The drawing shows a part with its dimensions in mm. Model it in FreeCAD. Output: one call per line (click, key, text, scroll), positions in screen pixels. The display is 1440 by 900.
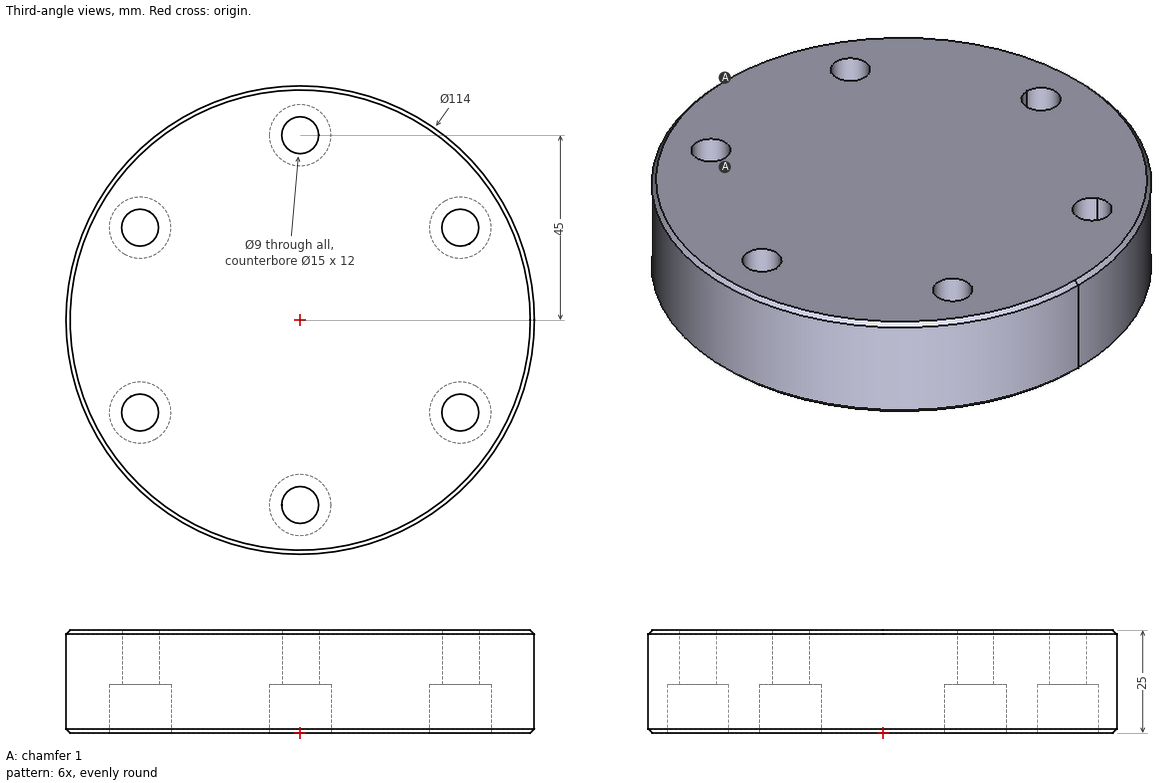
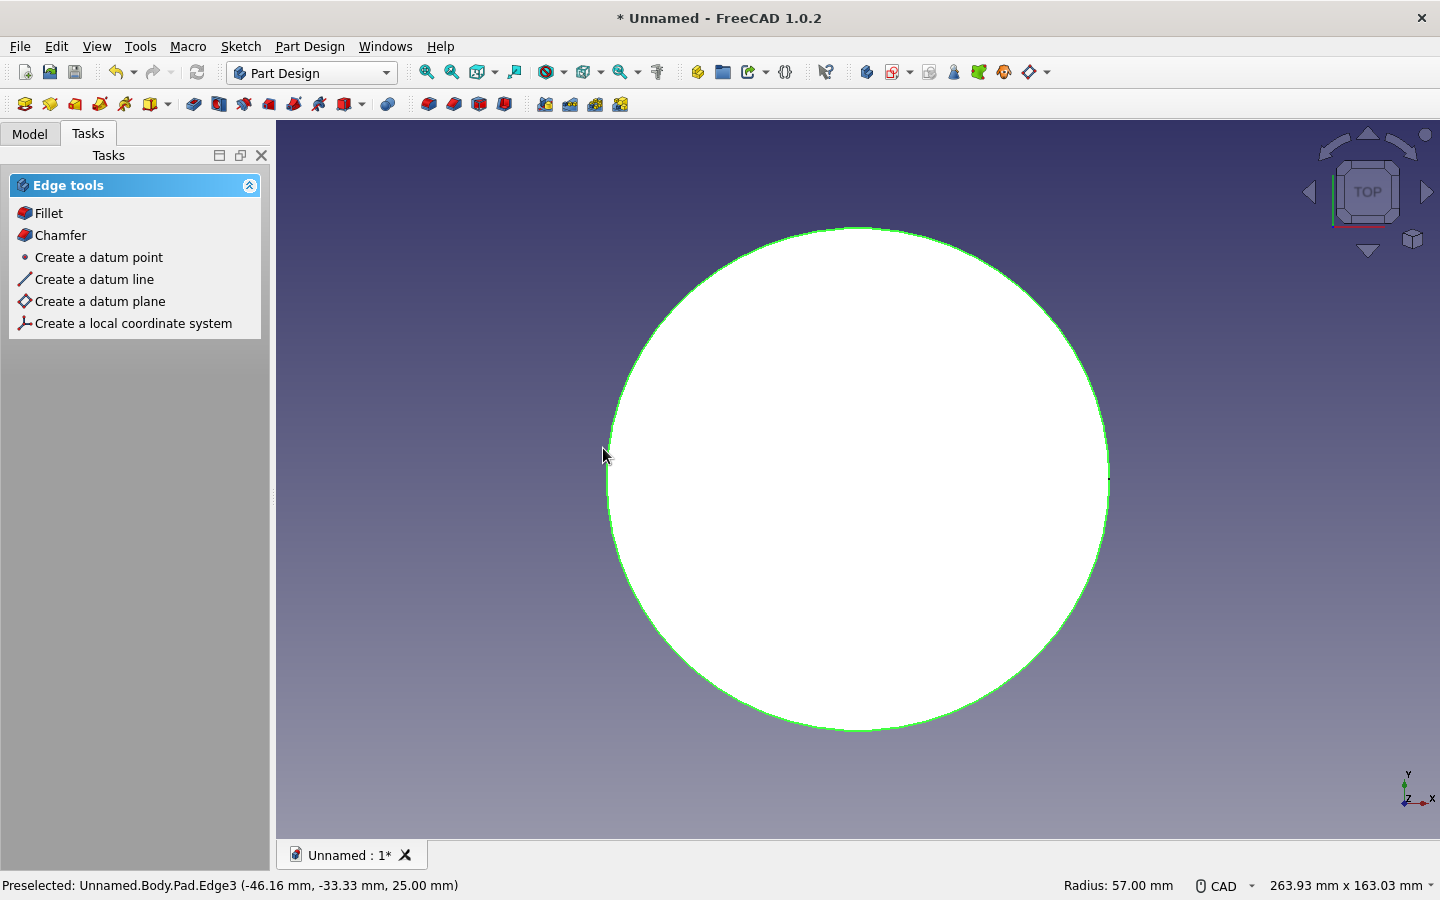
key(1)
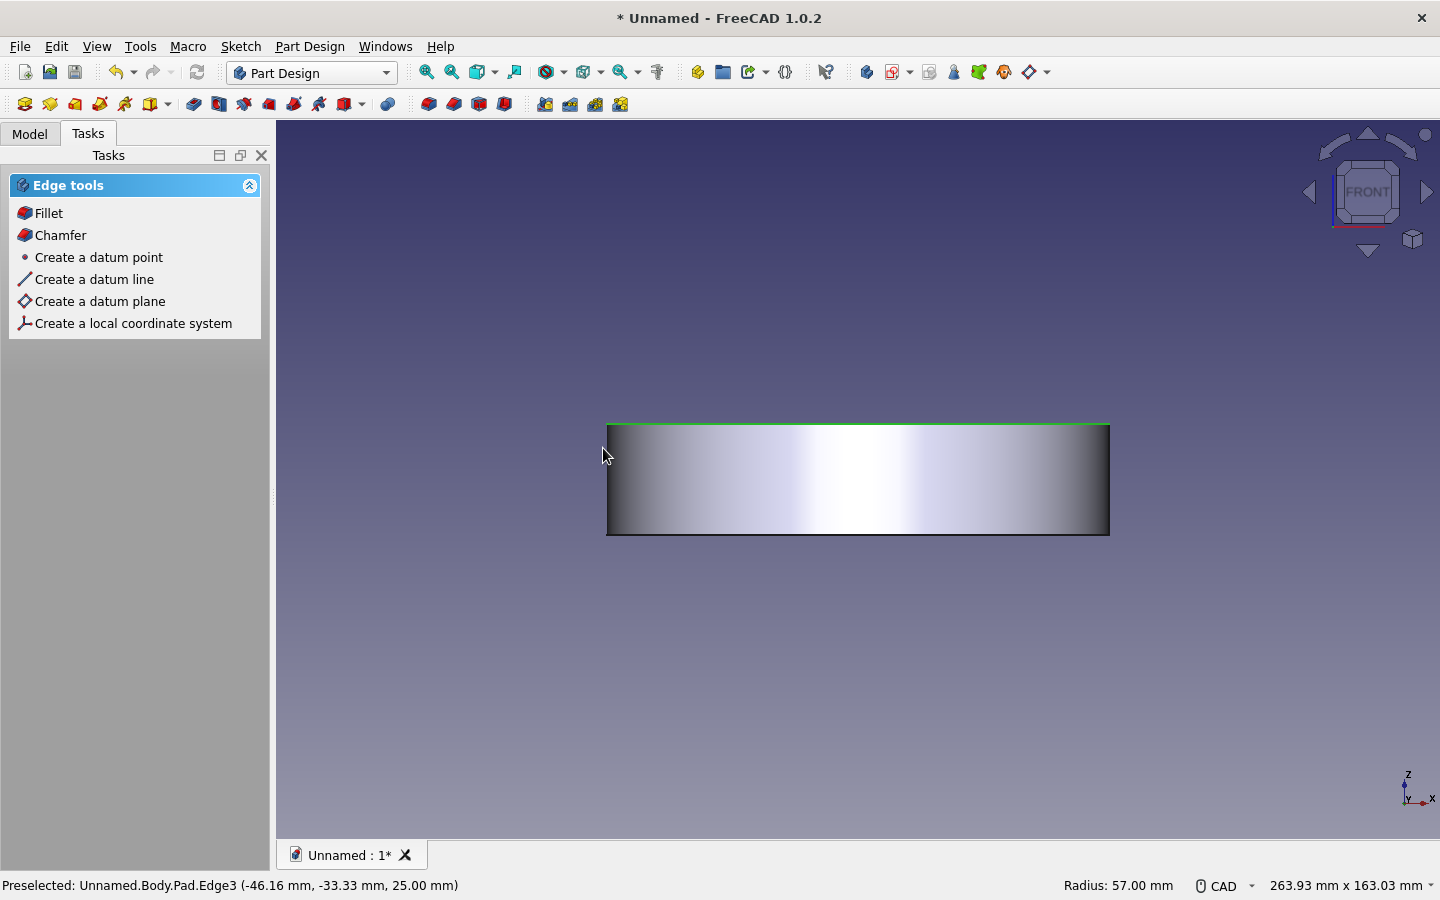
key(v)
key(f)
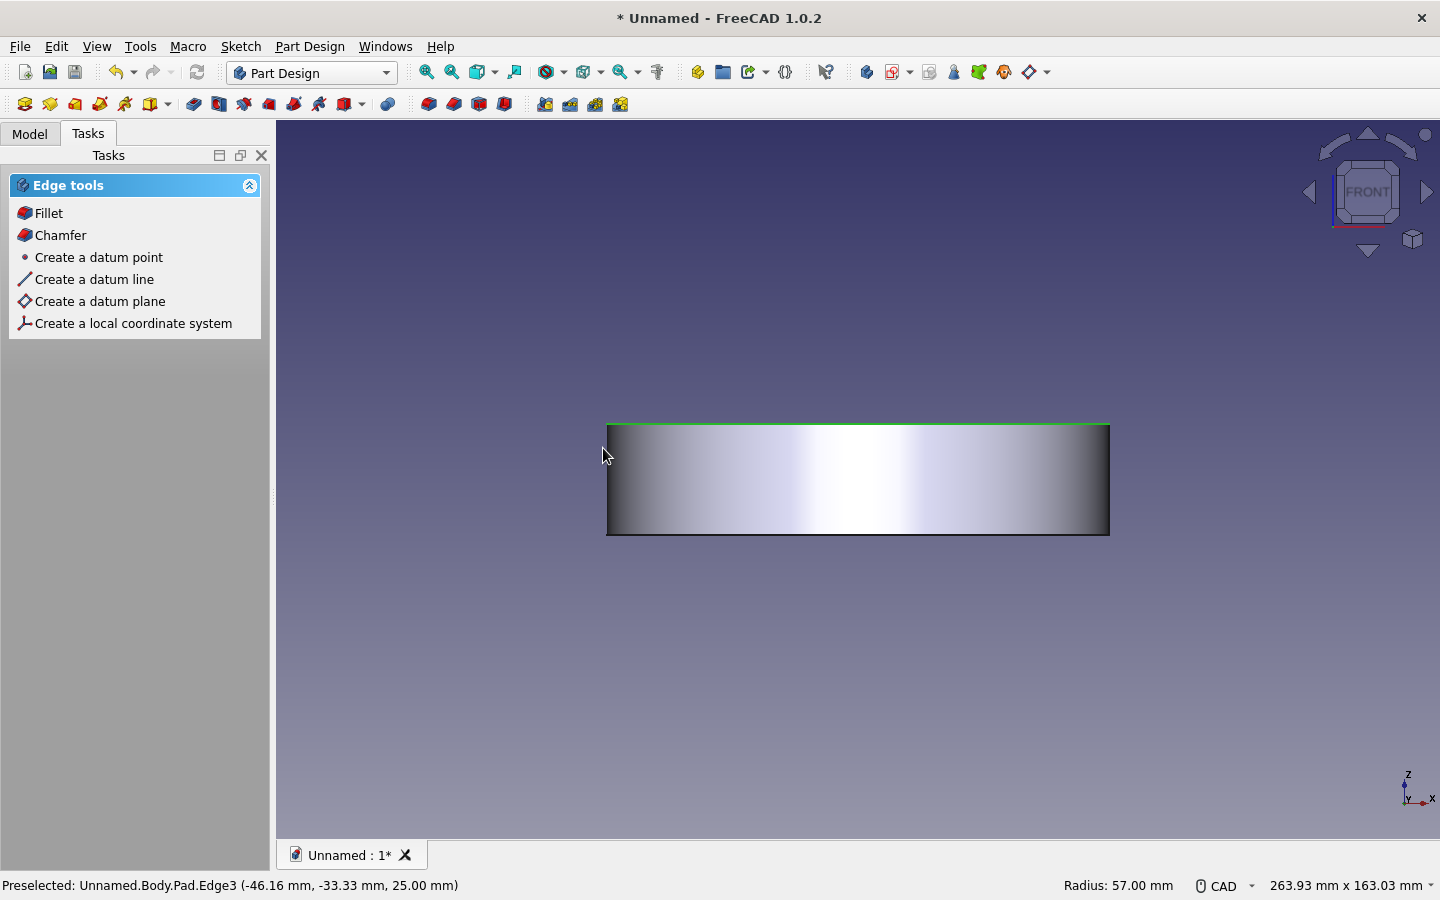
click(655, 534, ctrl)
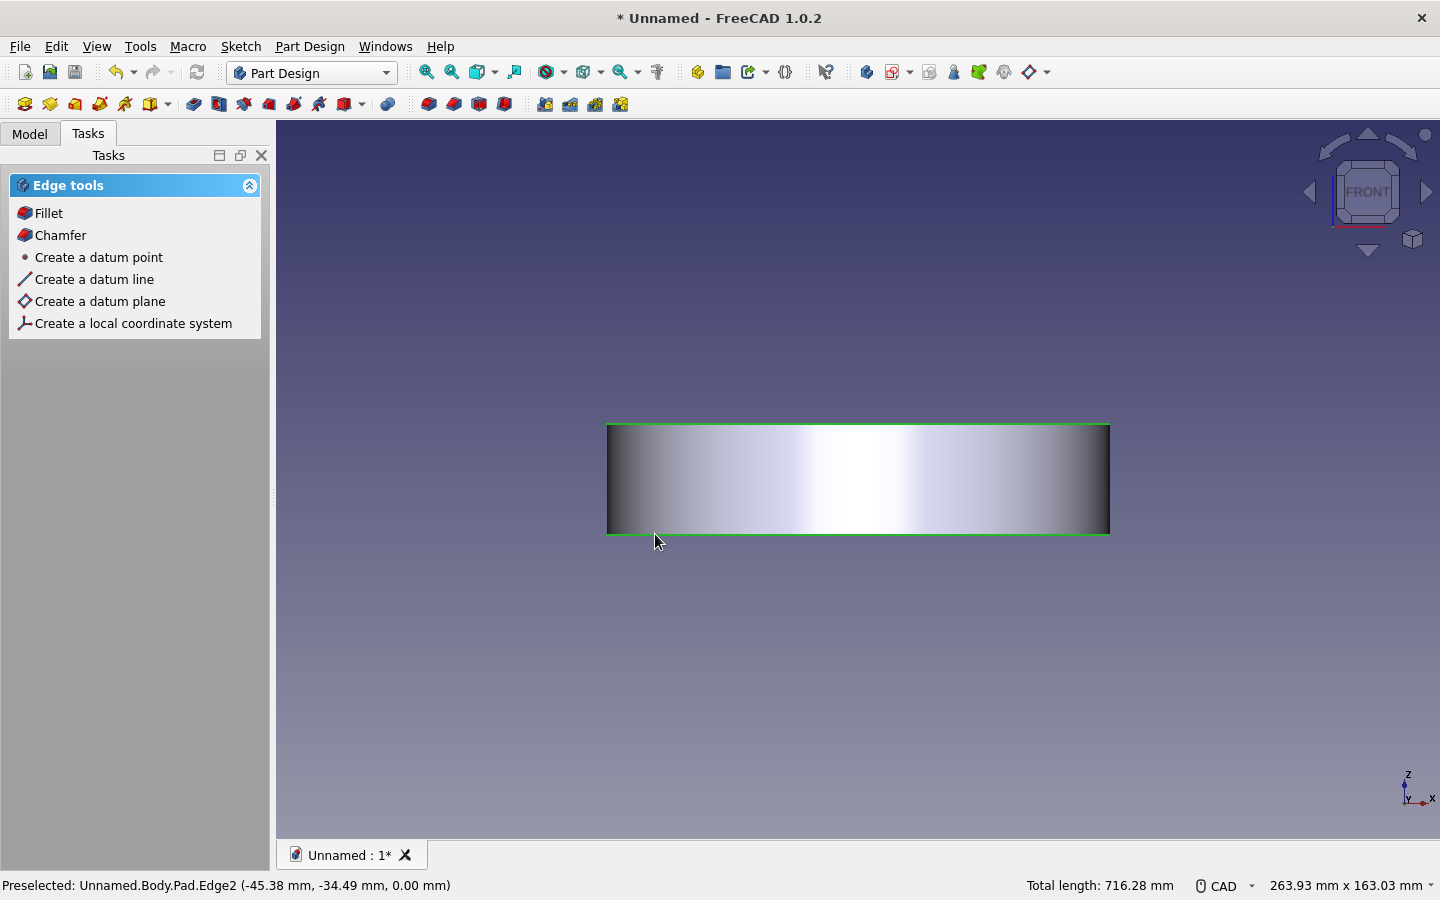
click(454, 104)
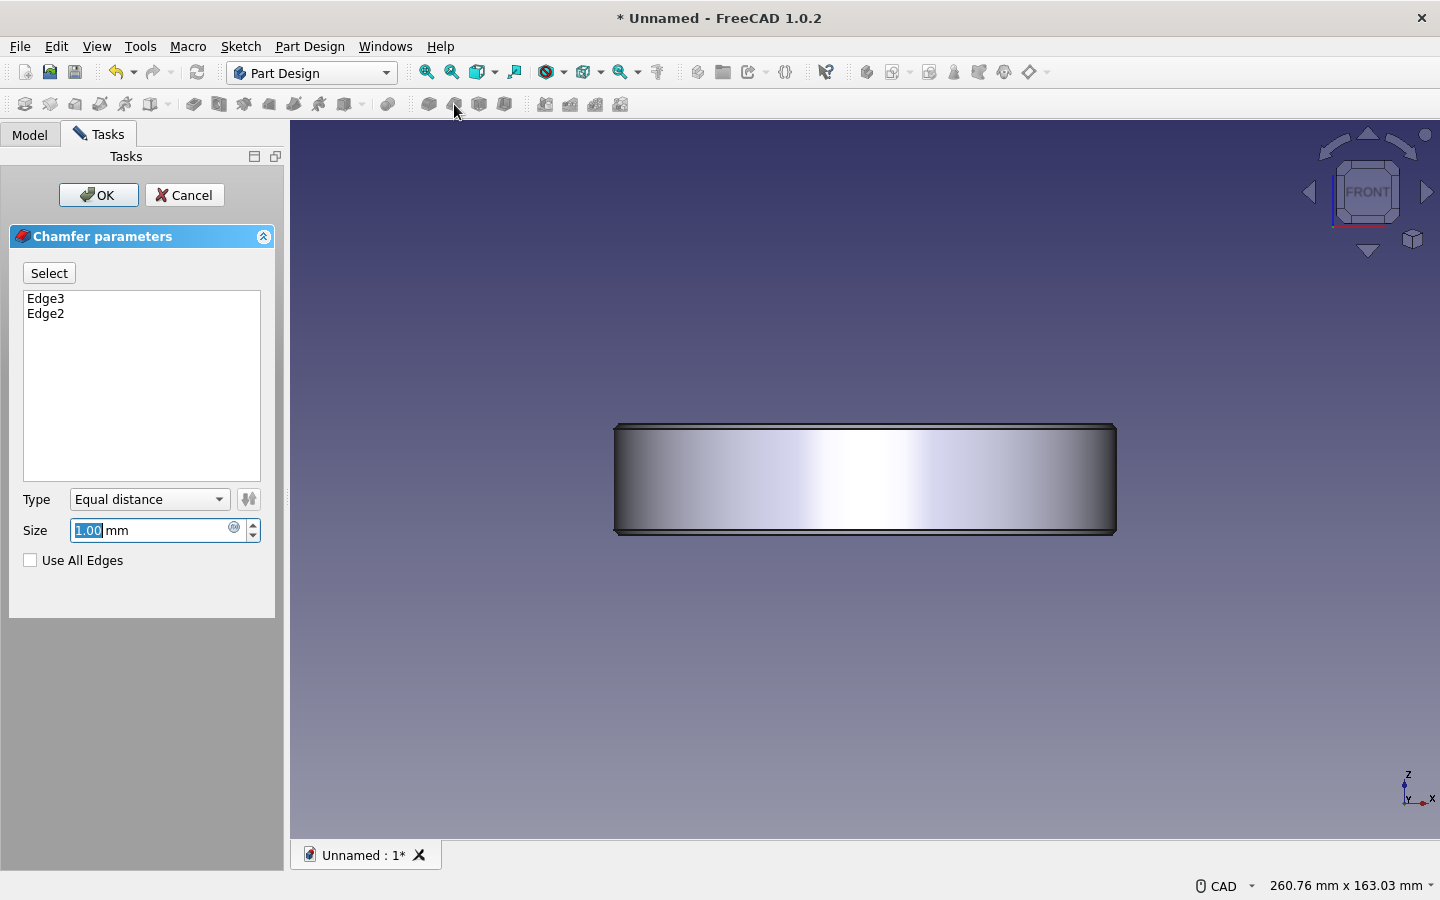
text(1)
key(Tab)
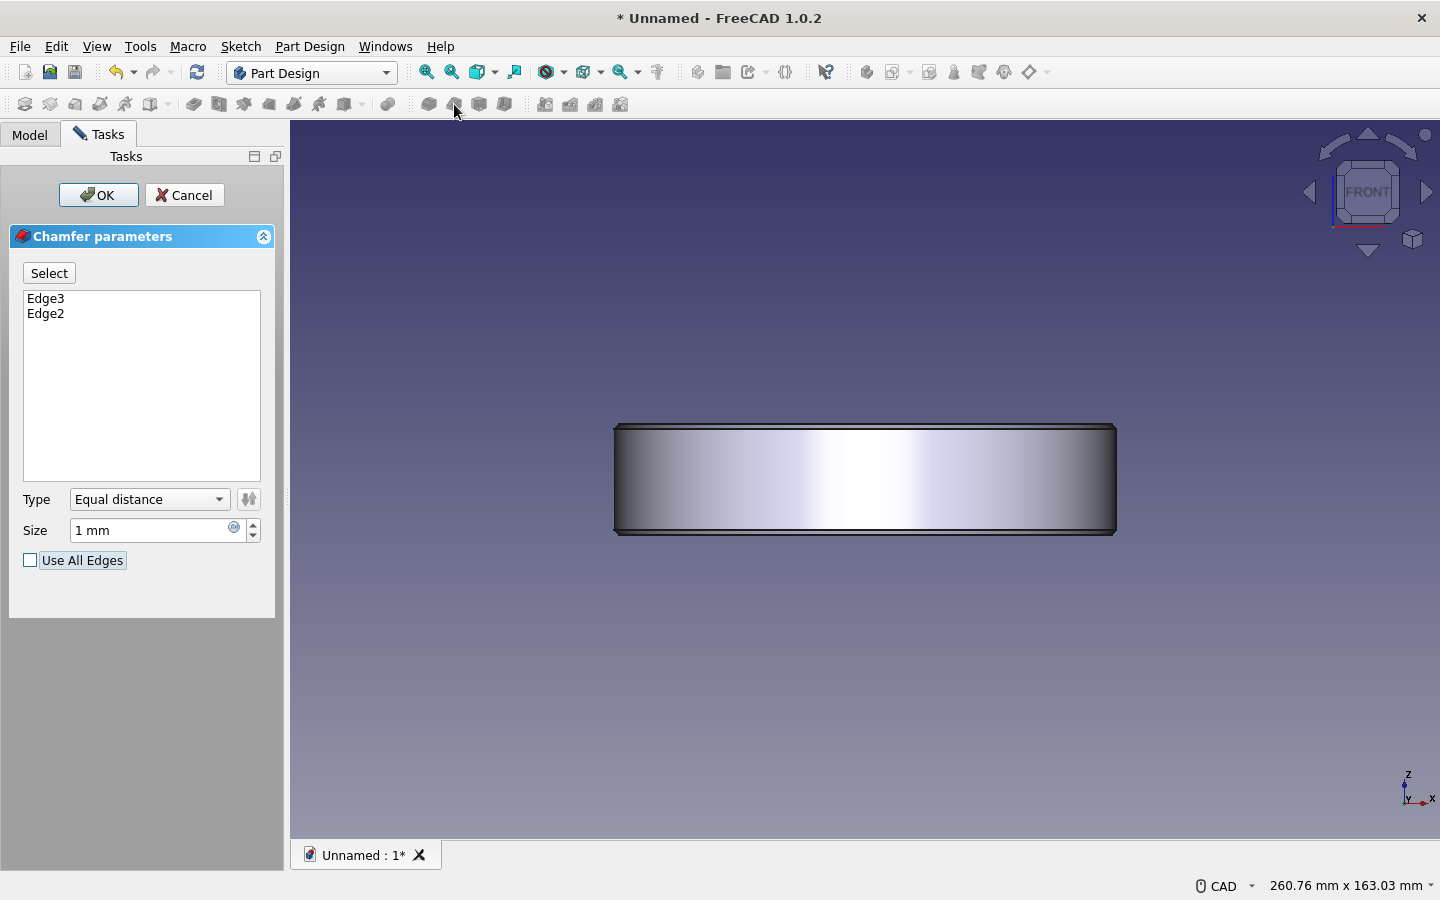
click(99, 195)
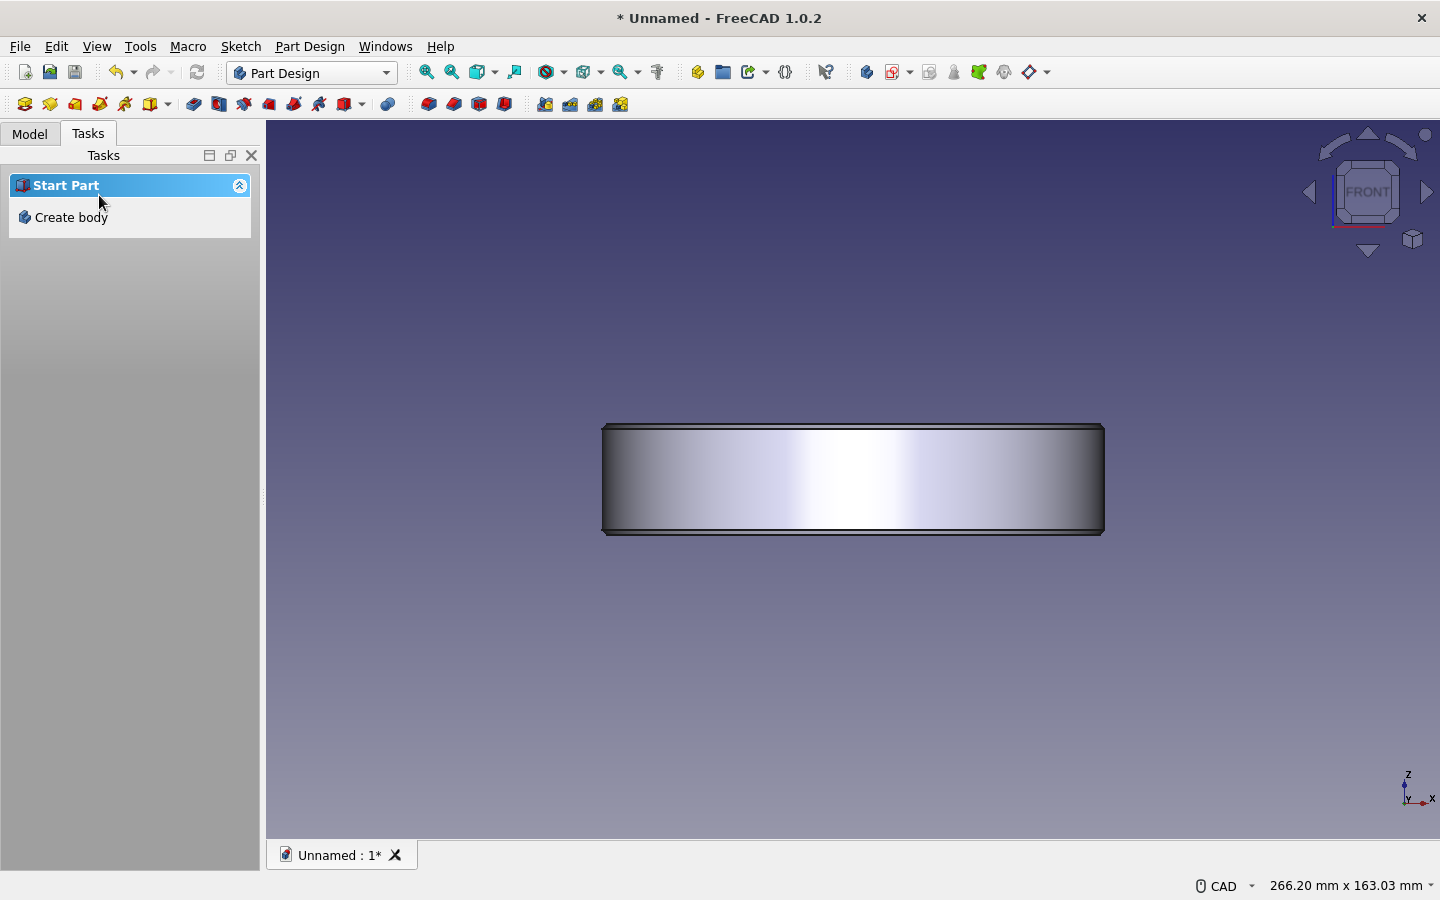
click(427, 72)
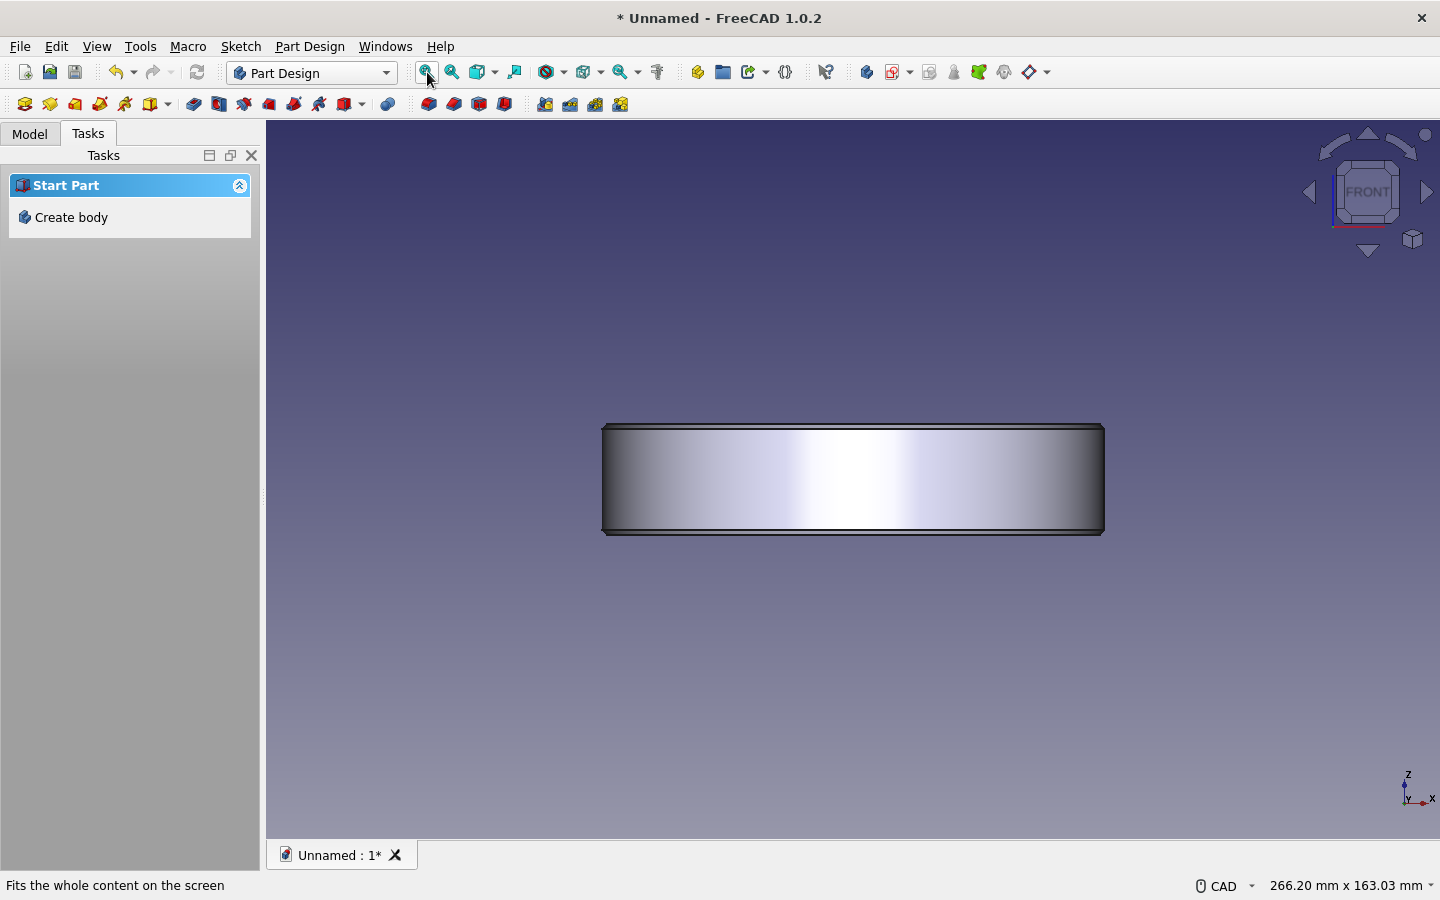
key(5)